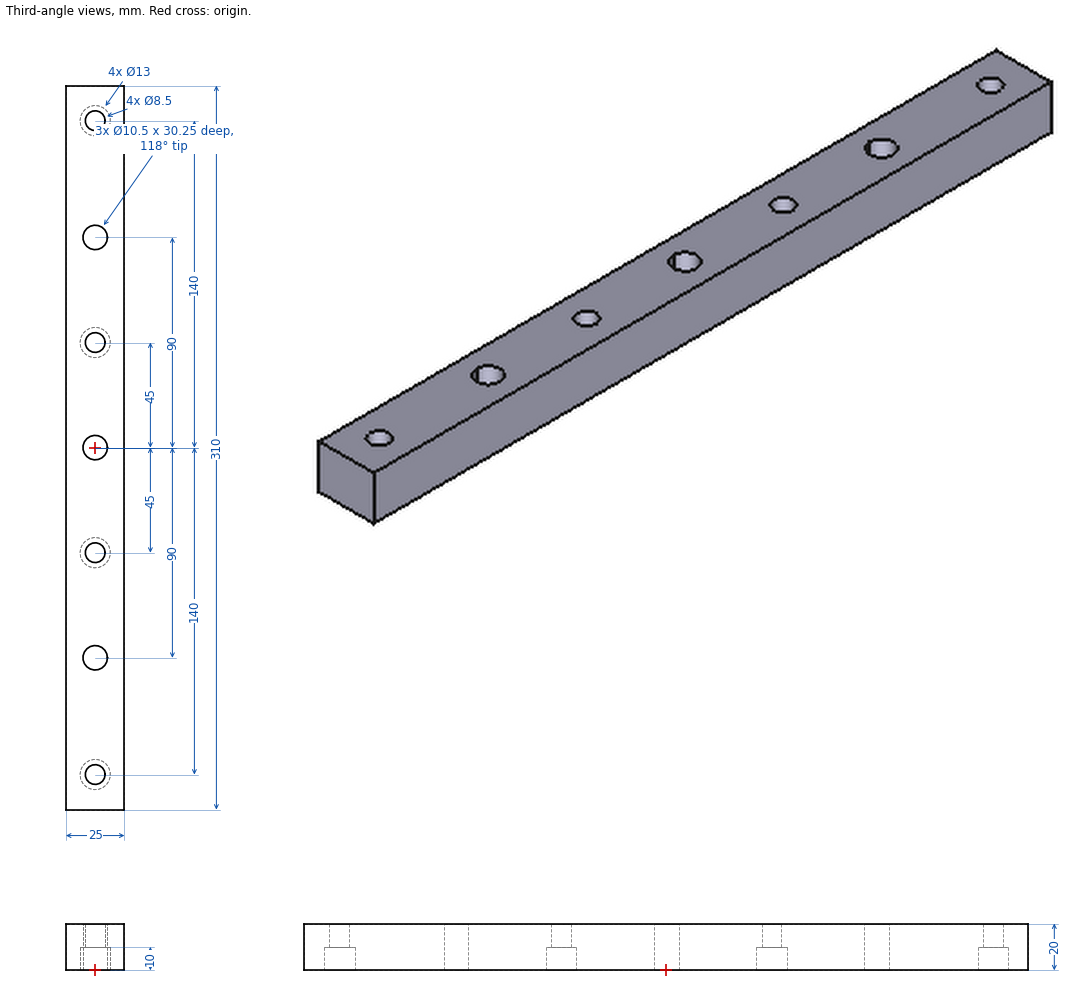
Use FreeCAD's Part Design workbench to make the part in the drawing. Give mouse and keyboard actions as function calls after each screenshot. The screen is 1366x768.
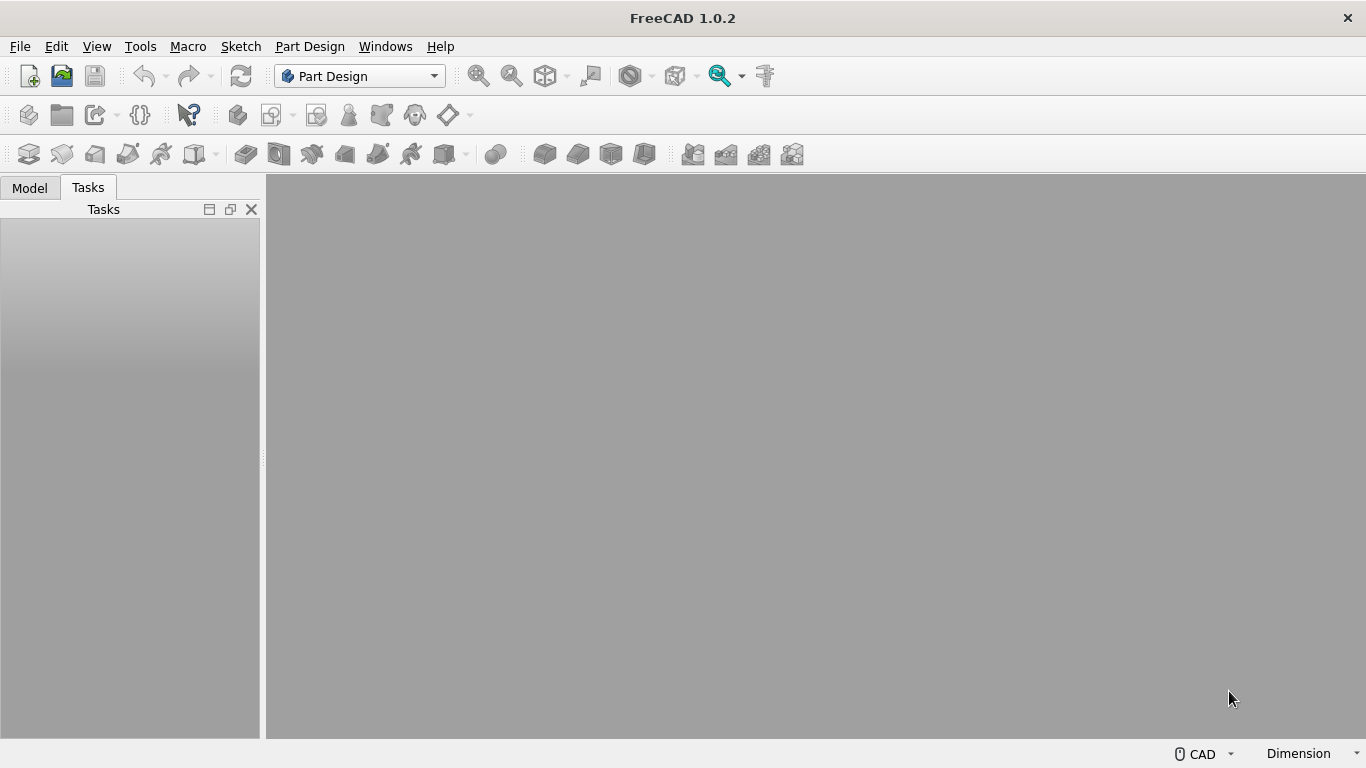
key(ctrl+n)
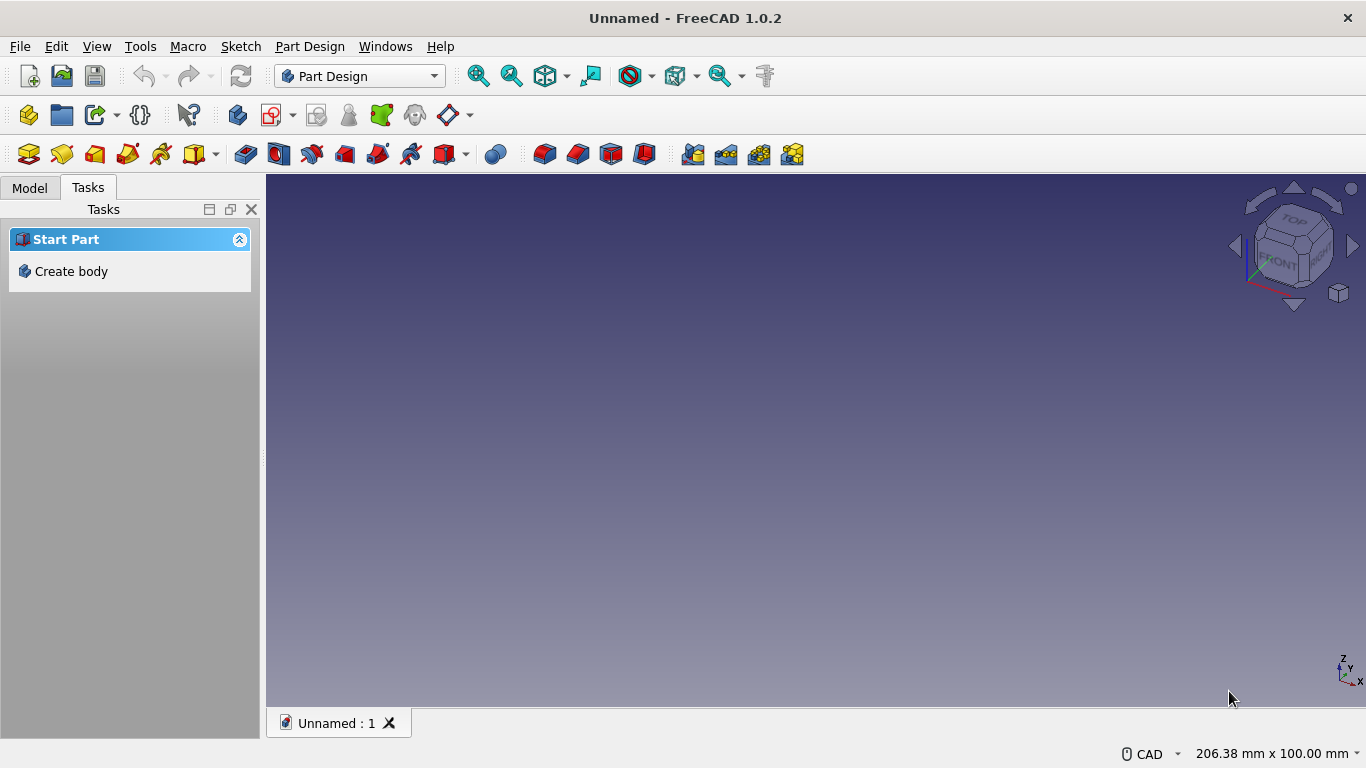
click(270, 116)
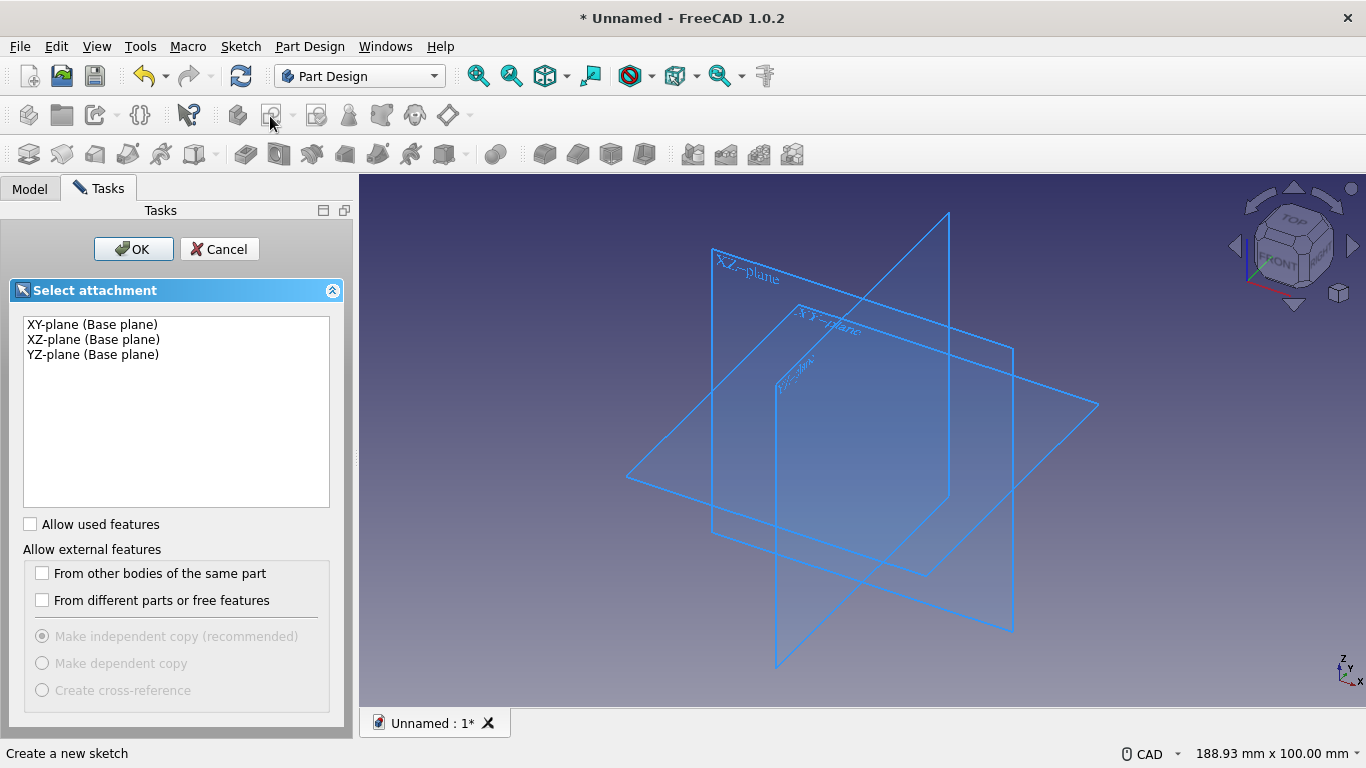
click(84, 324)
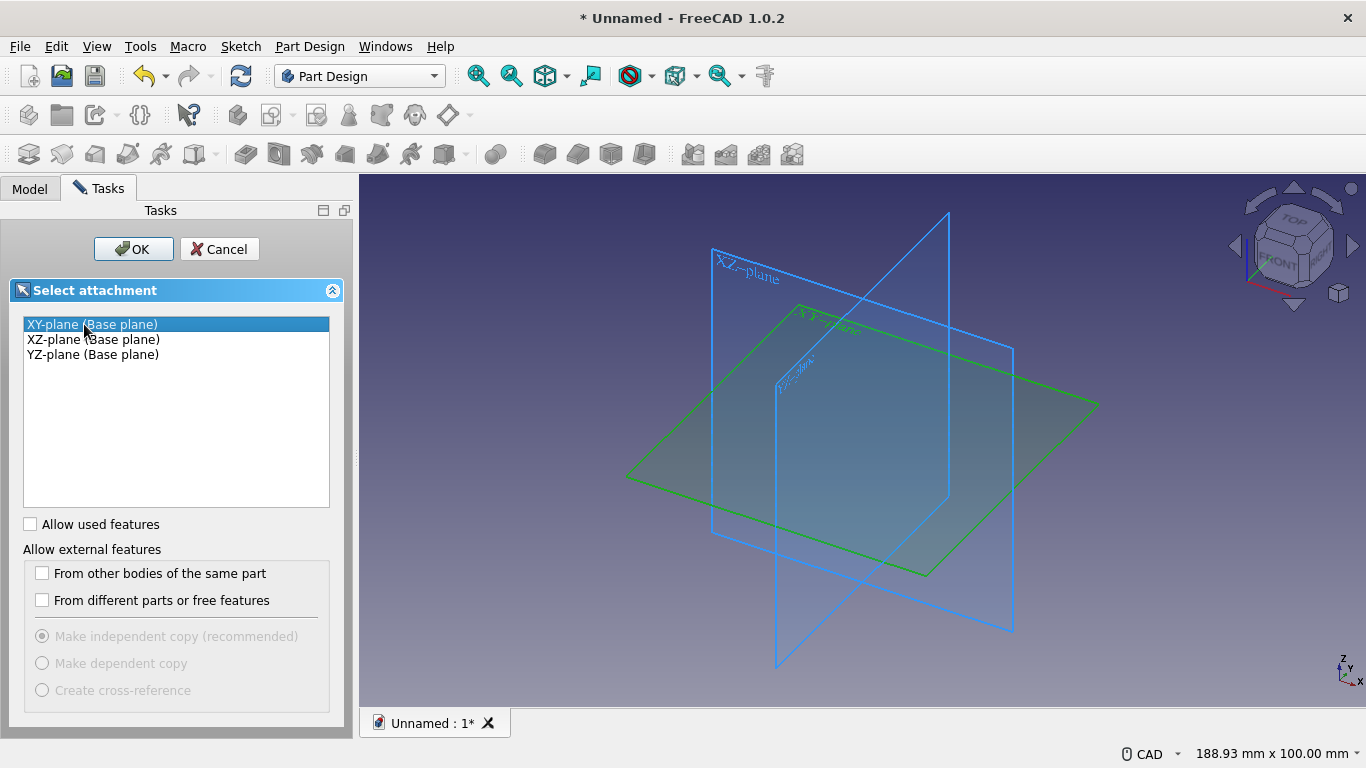
click(134, 249)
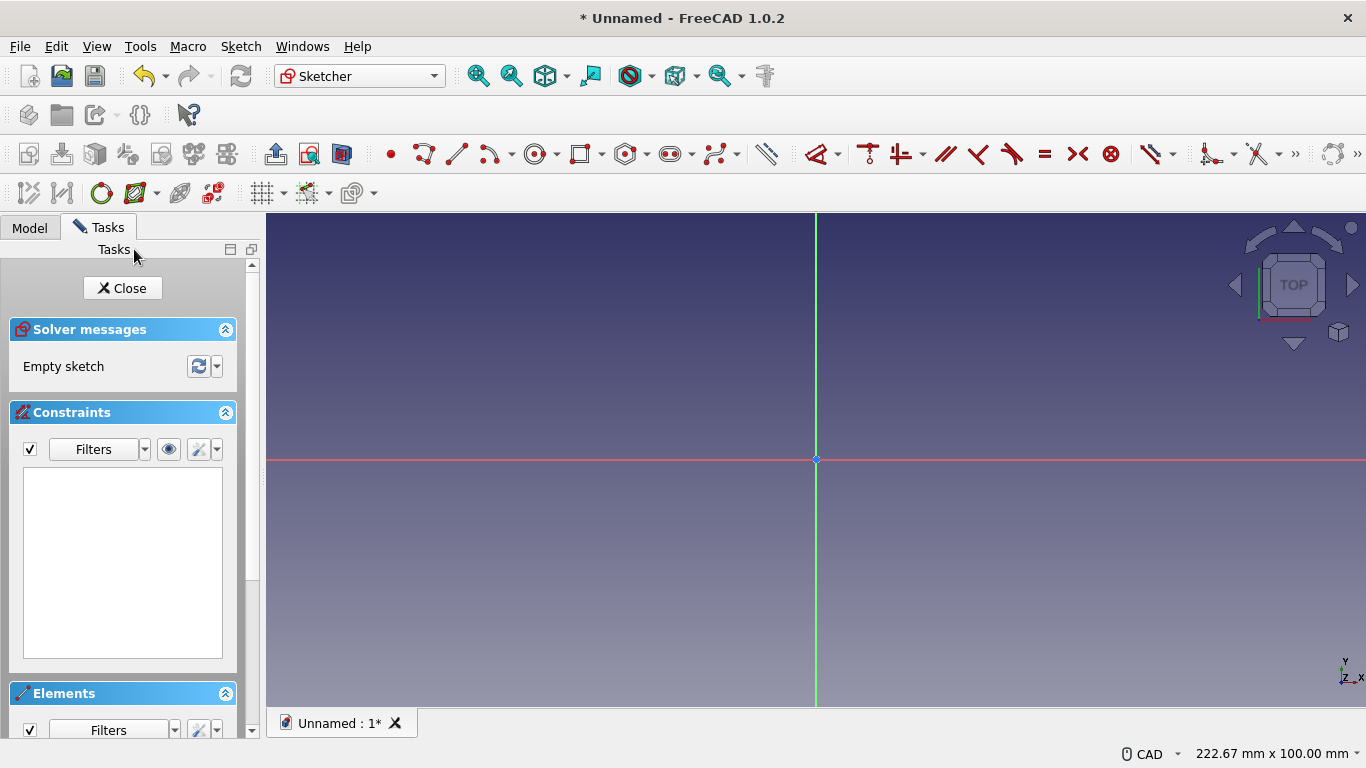
scroll(730, 460, down, 8)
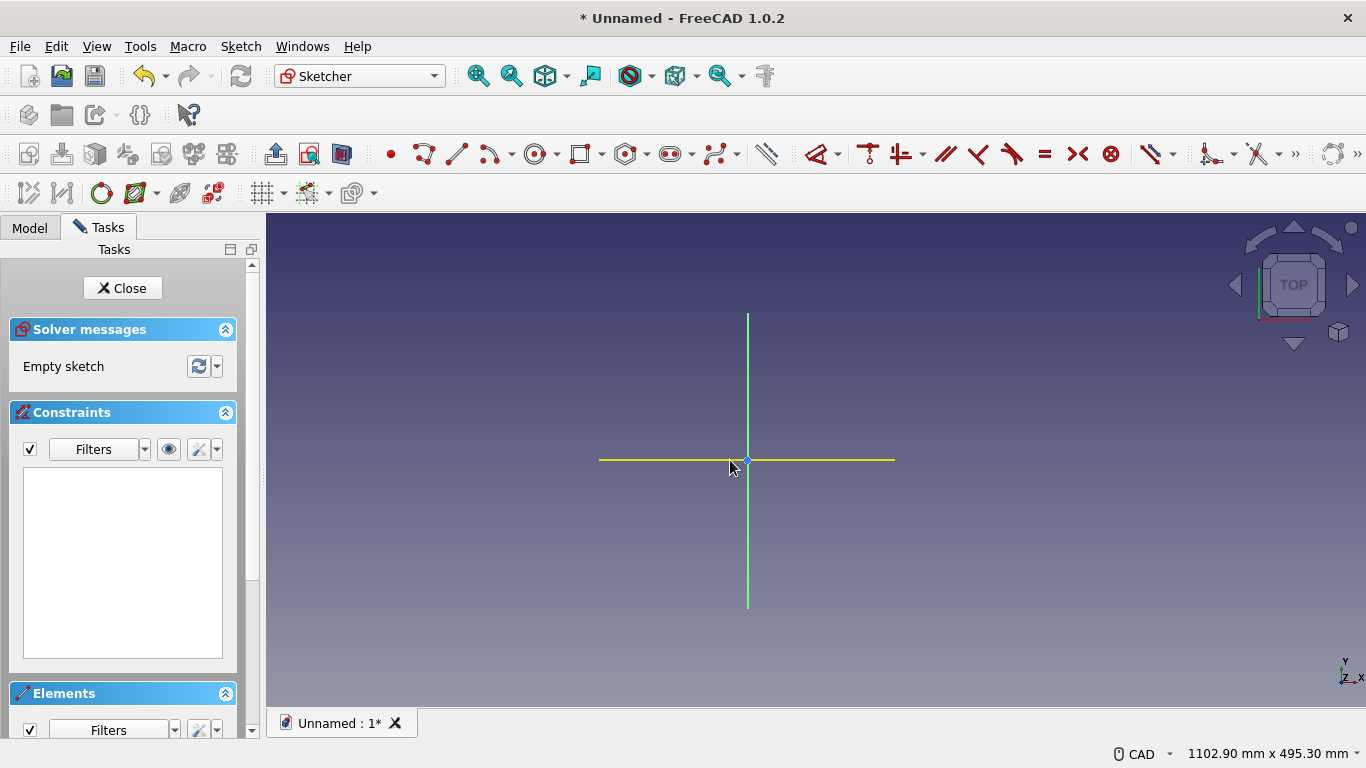
key(g)
key(v)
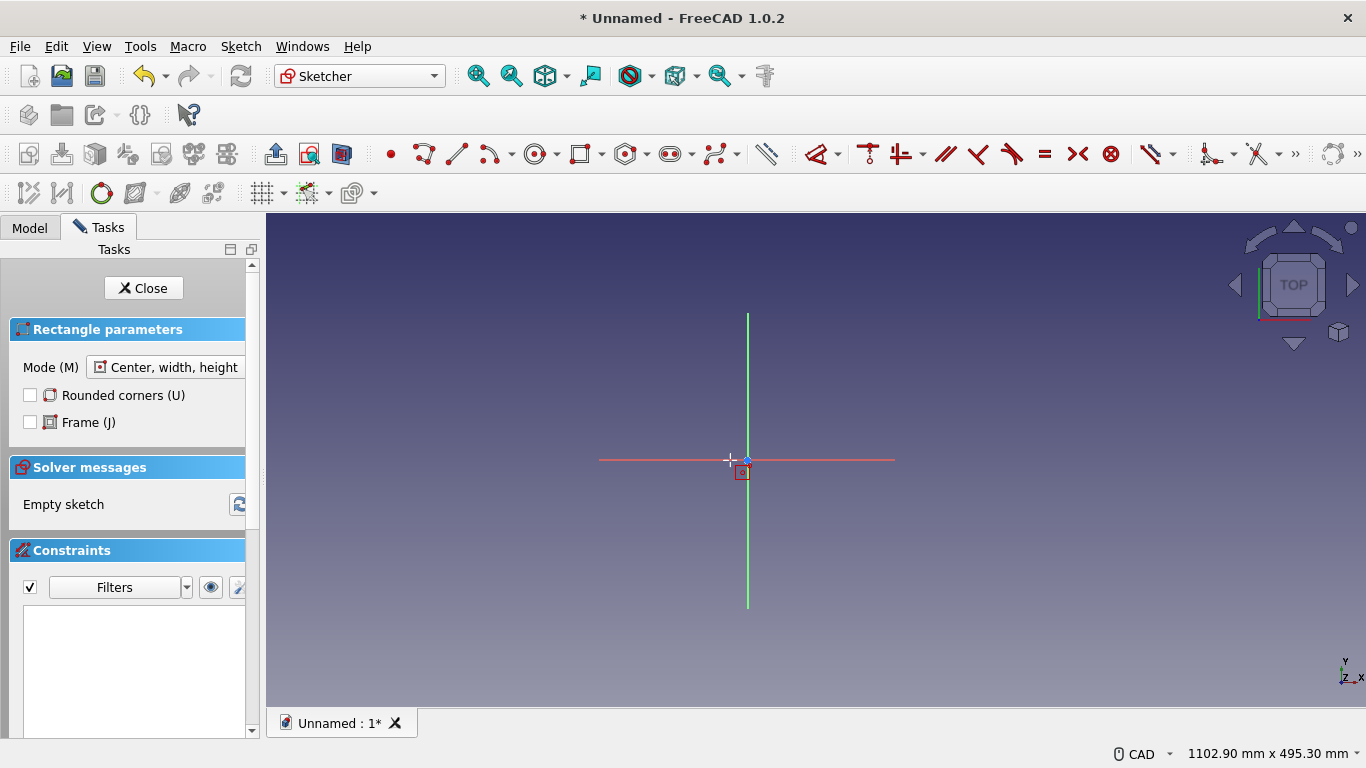
scroll(748, 460, up, 2)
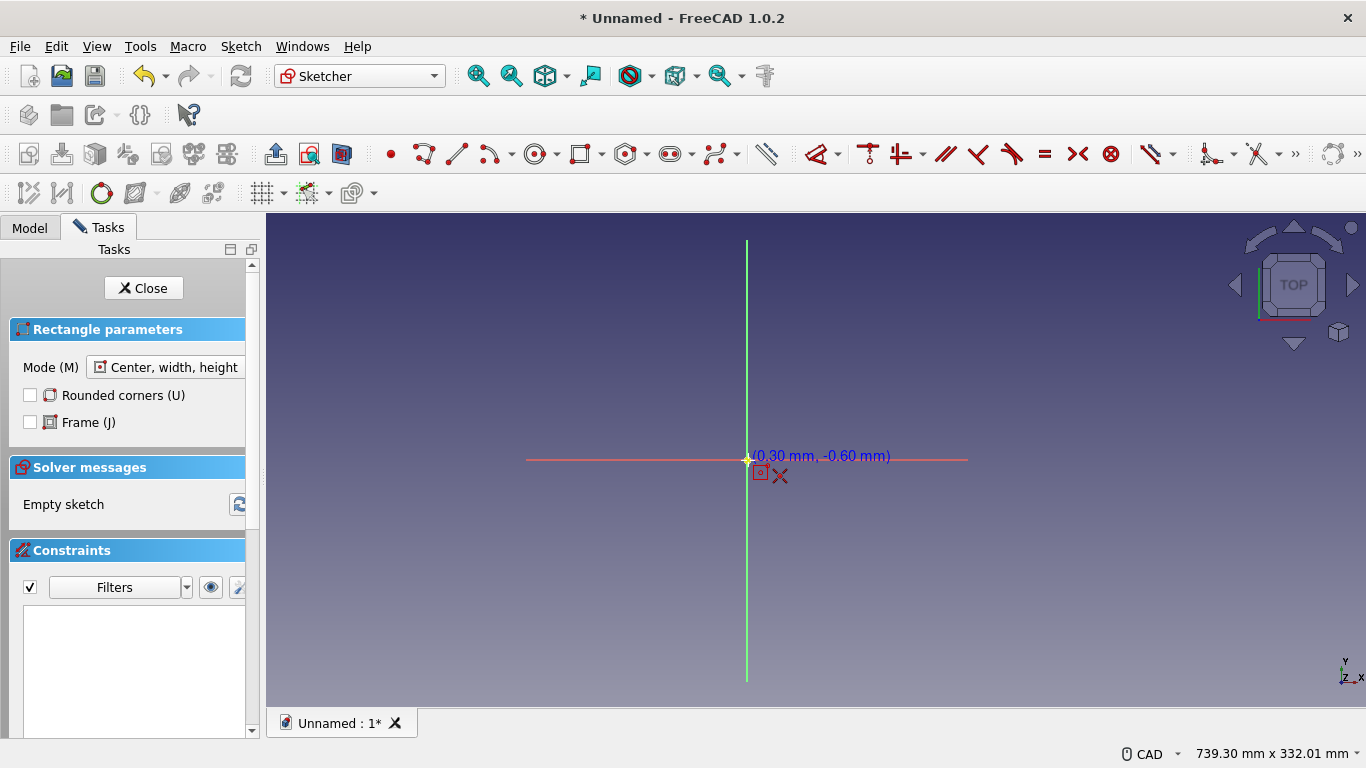
click(747, 460)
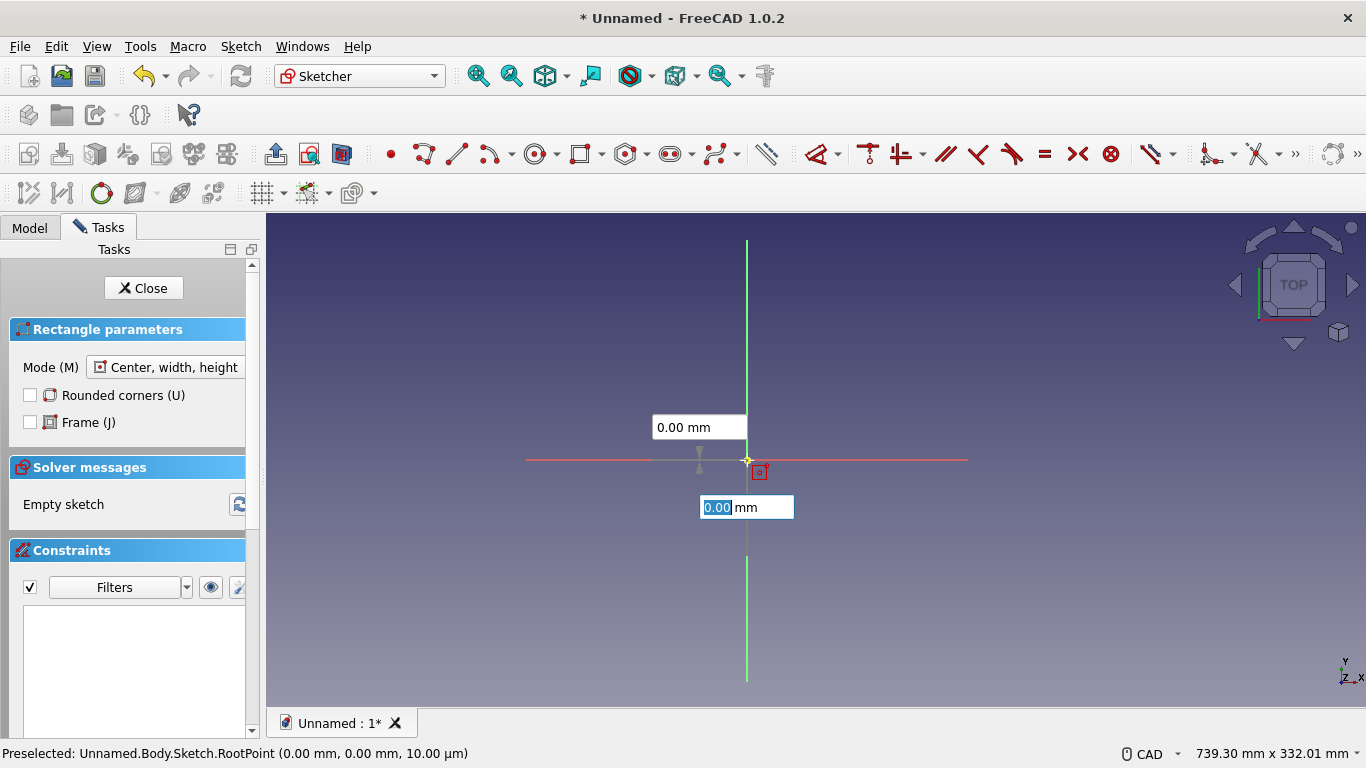
scroll(748, 459, down, 2)